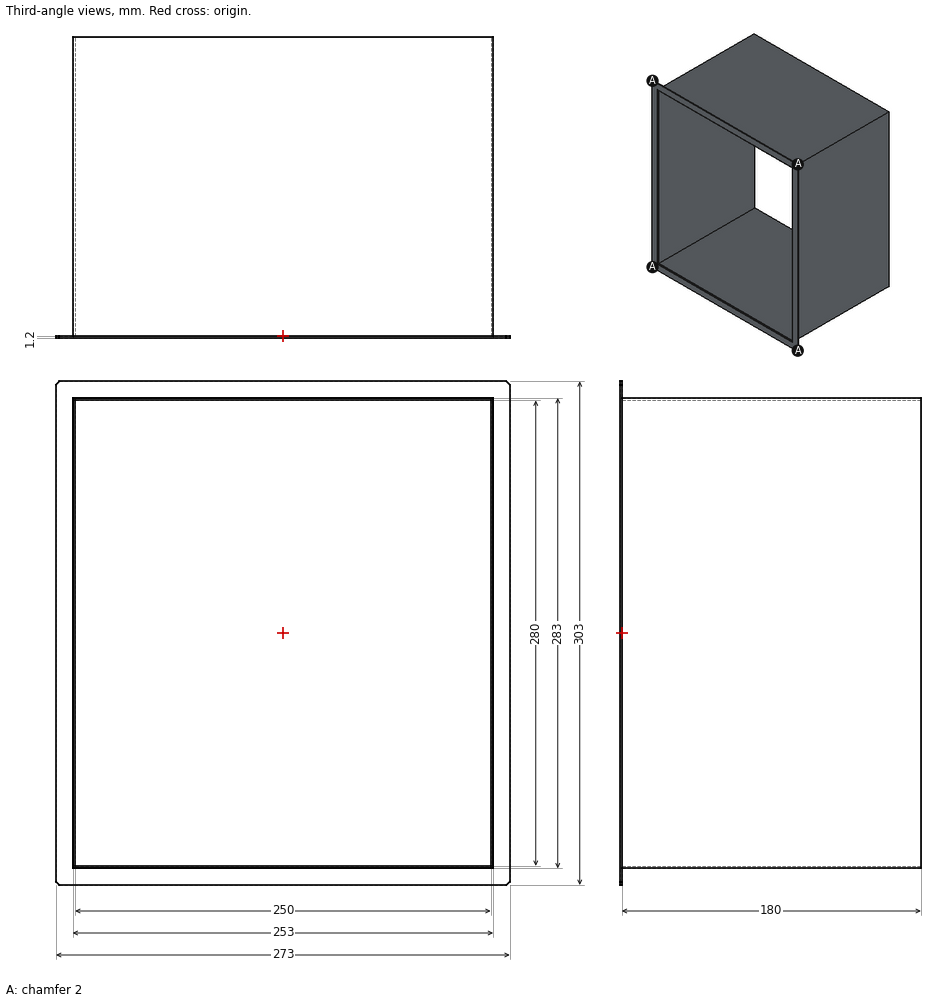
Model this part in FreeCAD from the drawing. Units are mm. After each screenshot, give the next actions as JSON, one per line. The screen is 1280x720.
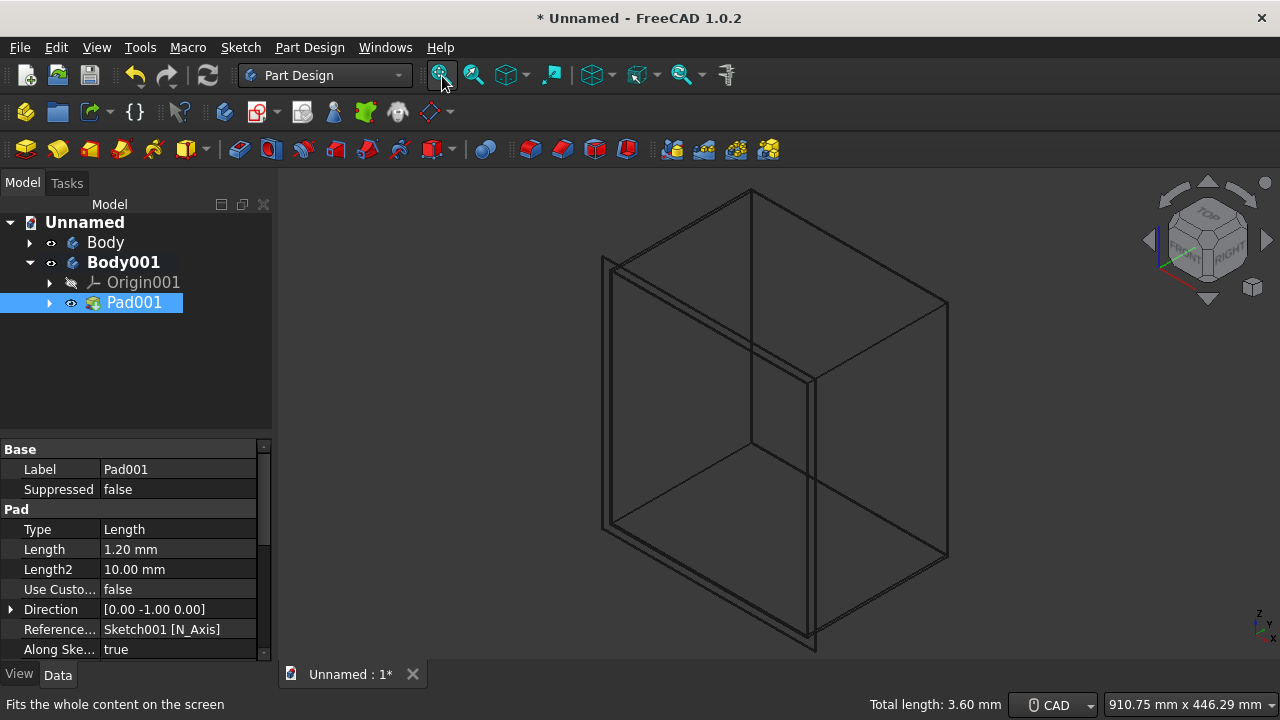
{"action": "scroll", "coordinate": [815, 378], "scroll_direction": "up", "scroll_amount": 15}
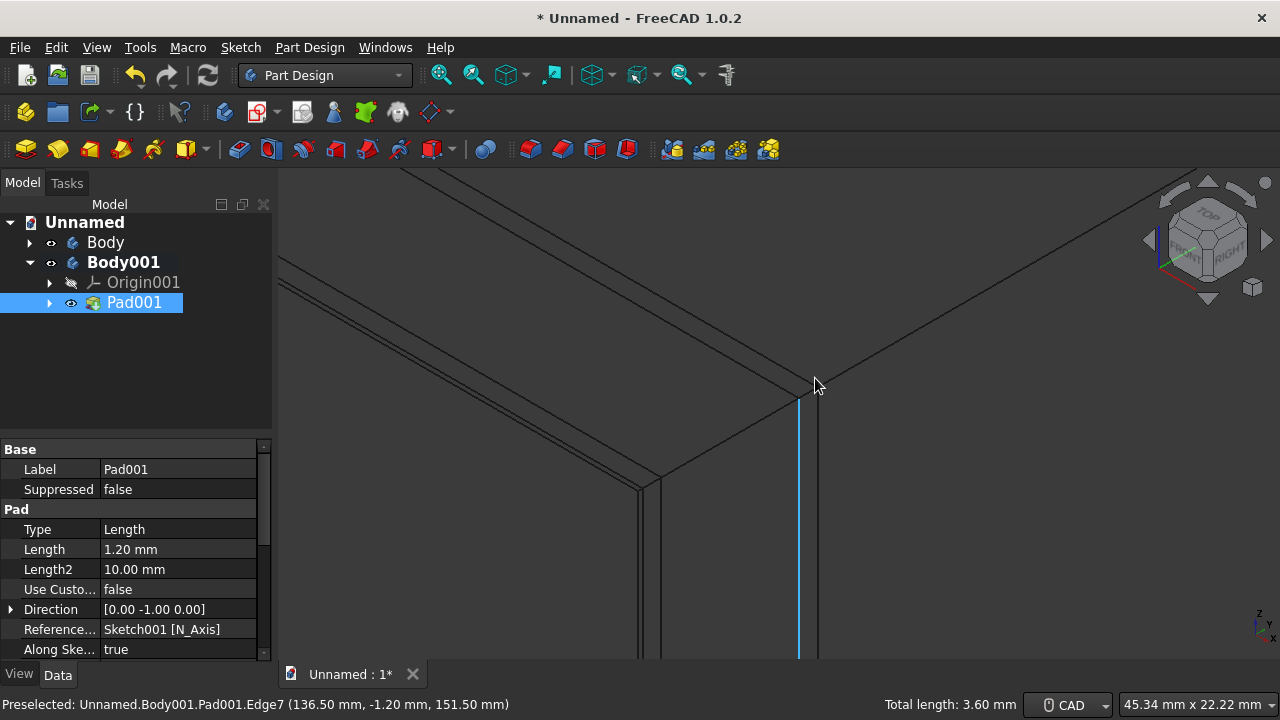
{"action": "left_click", "coordinate": [808, 392], "text": "ctrl"}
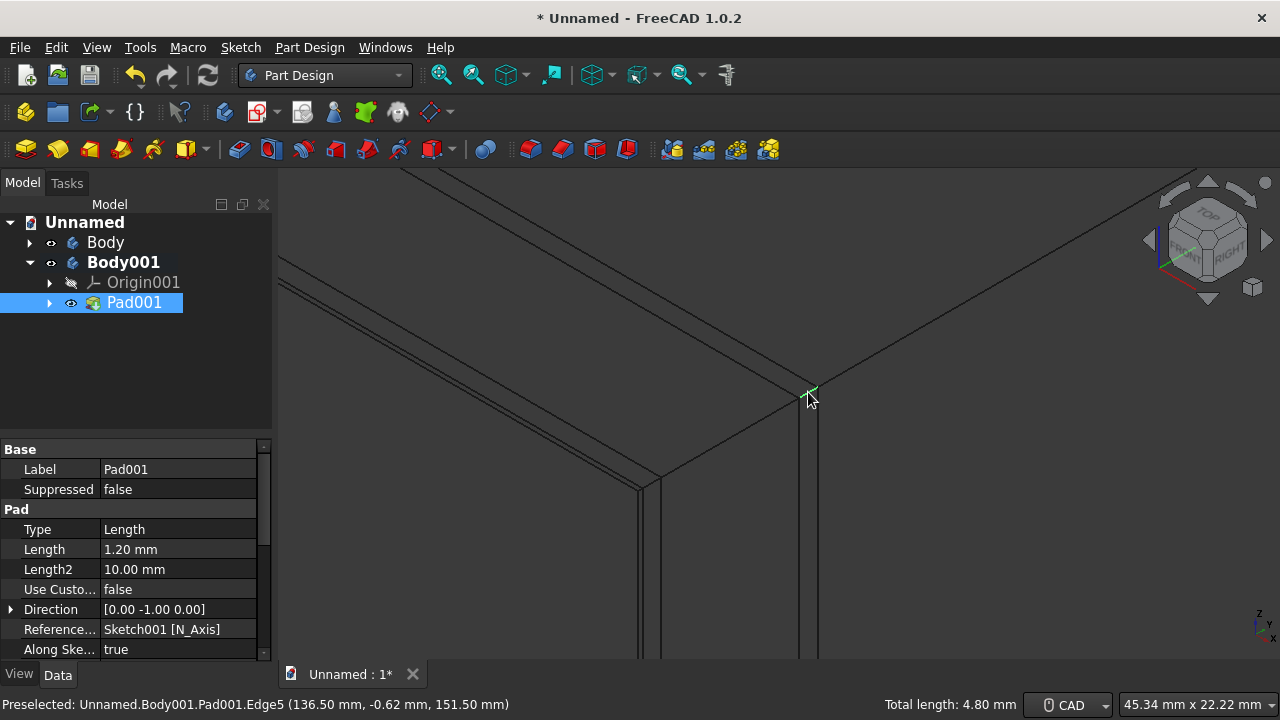
{"action": "key", "text": "v 1"}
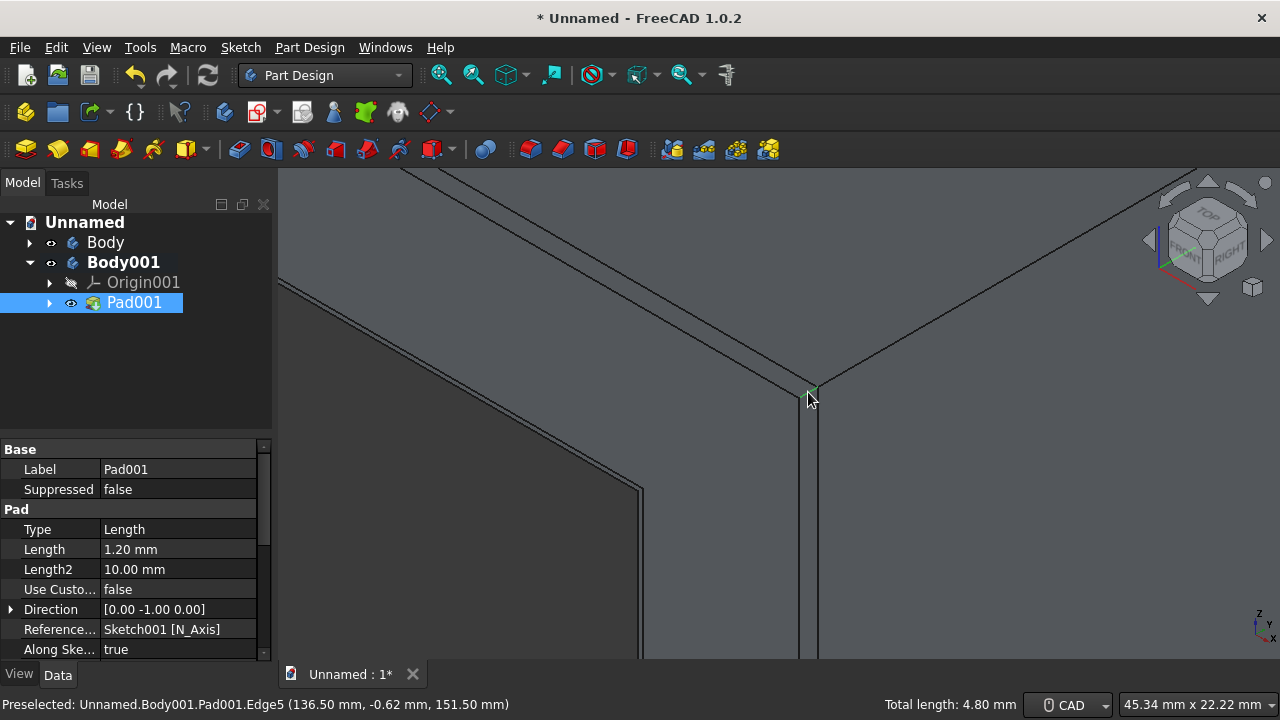
{"action": "left_click", "coordinate": [564, 150]}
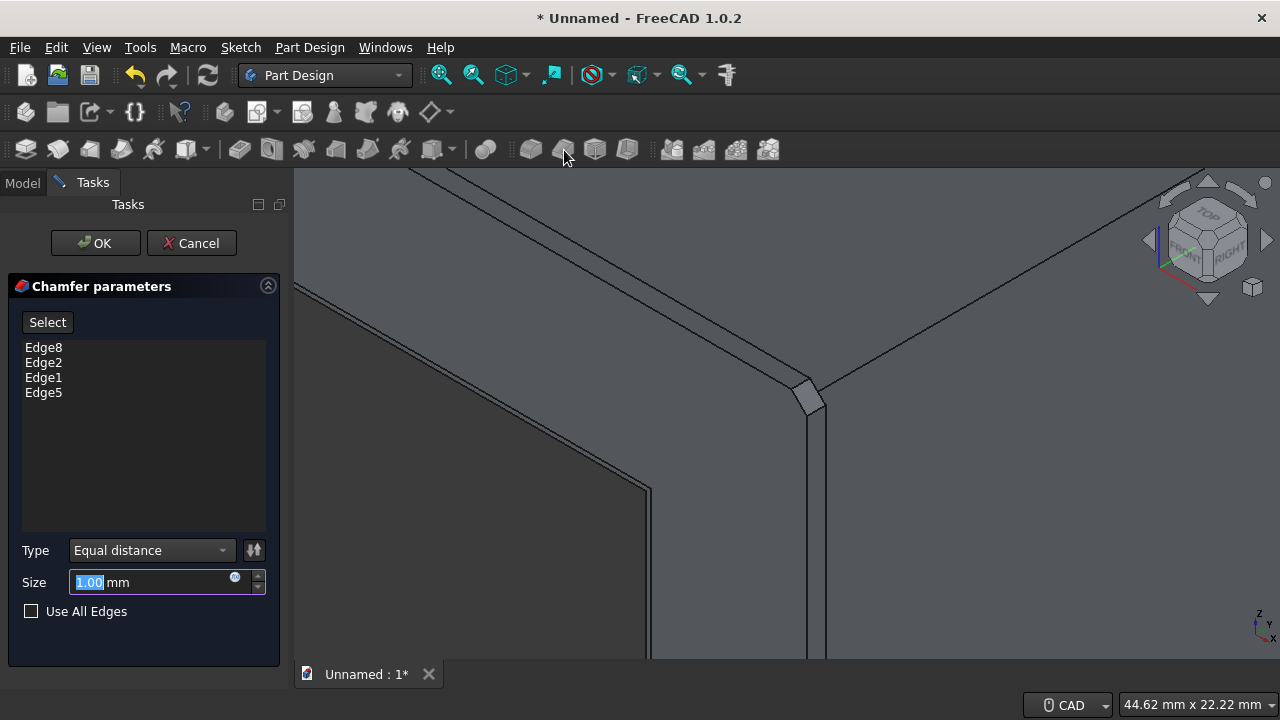
{"action": "type", "text": "2"}
{"action": "key", "text": "Tab"}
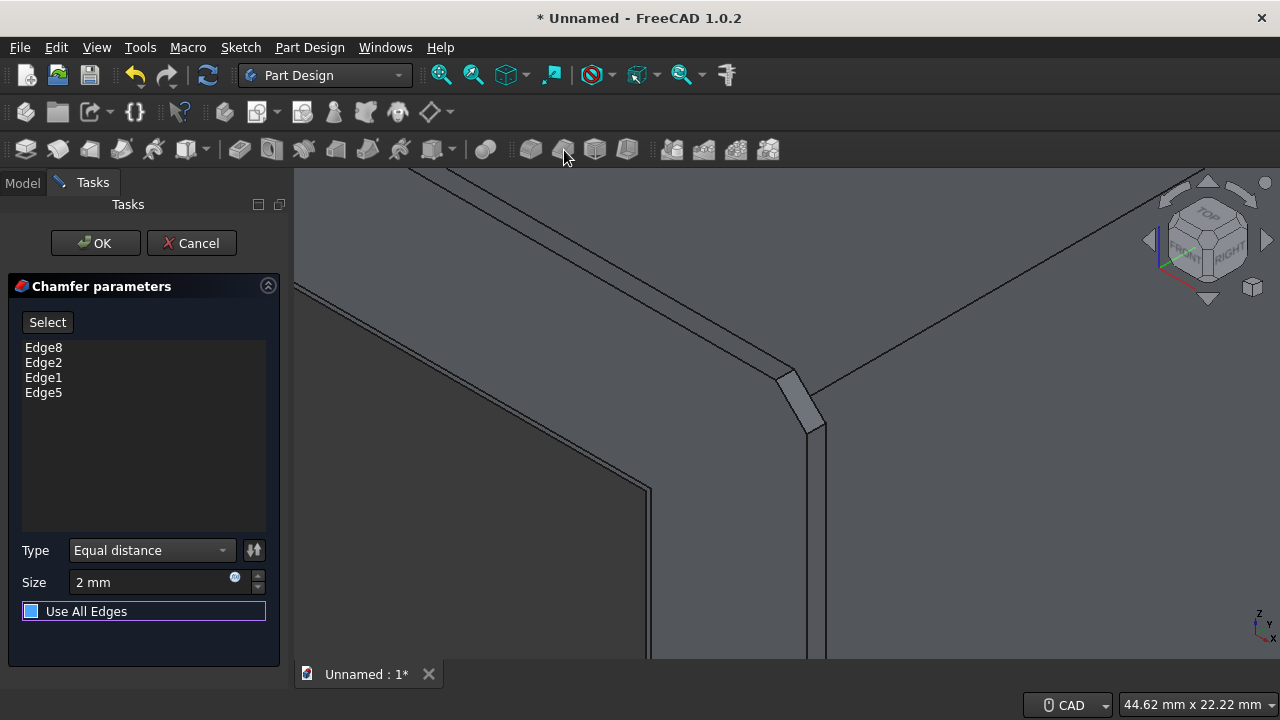
{"action": "left_click", "coordinate": [96, 243]}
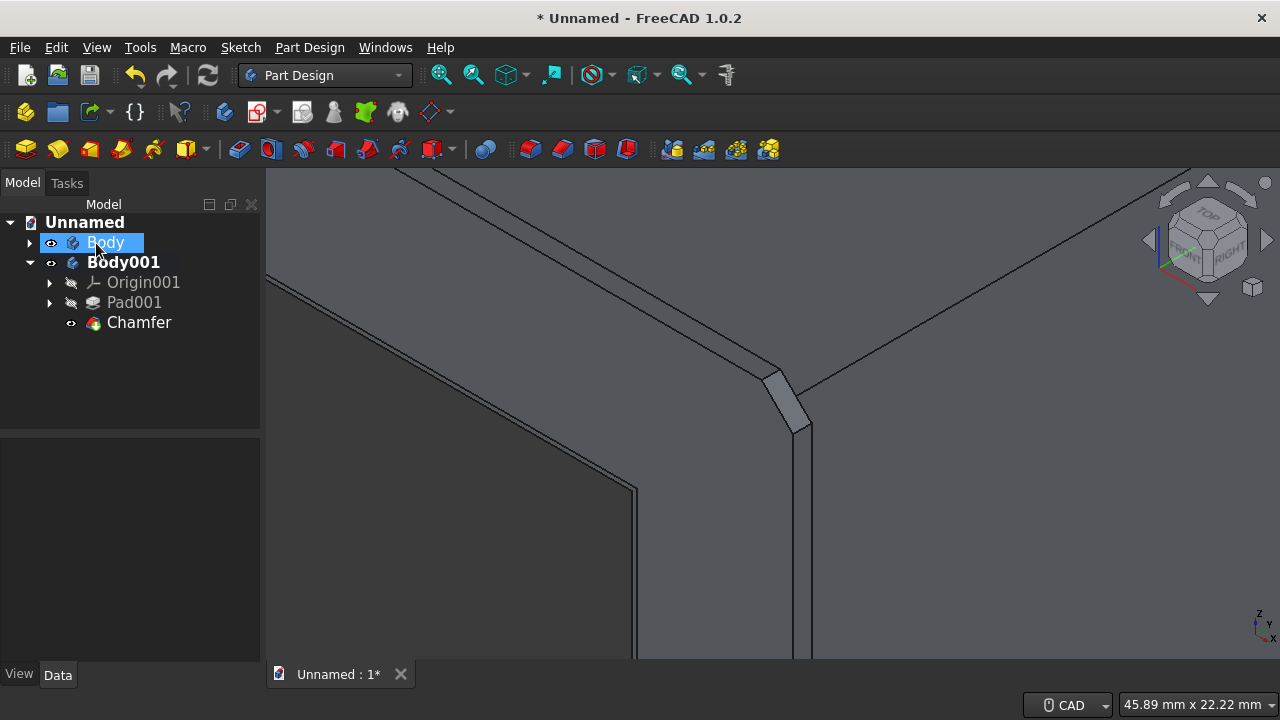
{"action": "left_click", "coordinate": [442, 76]}